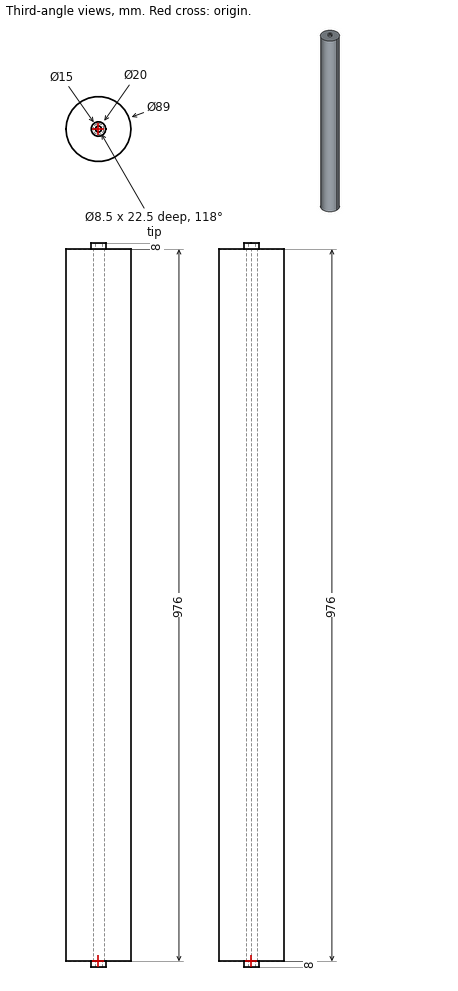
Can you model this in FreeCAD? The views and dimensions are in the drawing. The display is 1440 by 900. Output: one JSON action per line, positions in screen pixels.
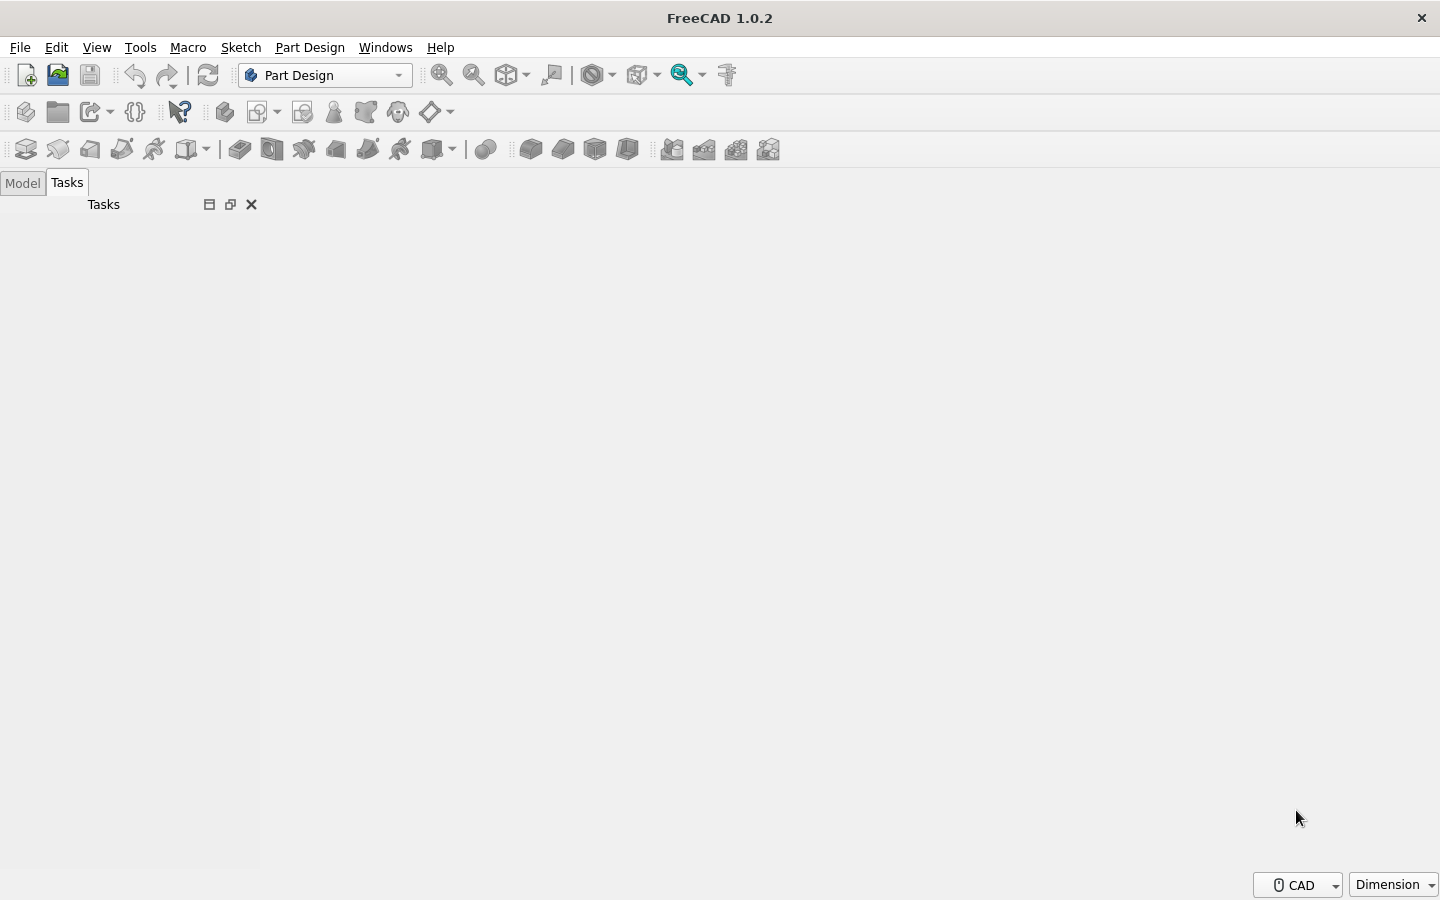
{"action": "left_click", "coordinate": [26, 76]}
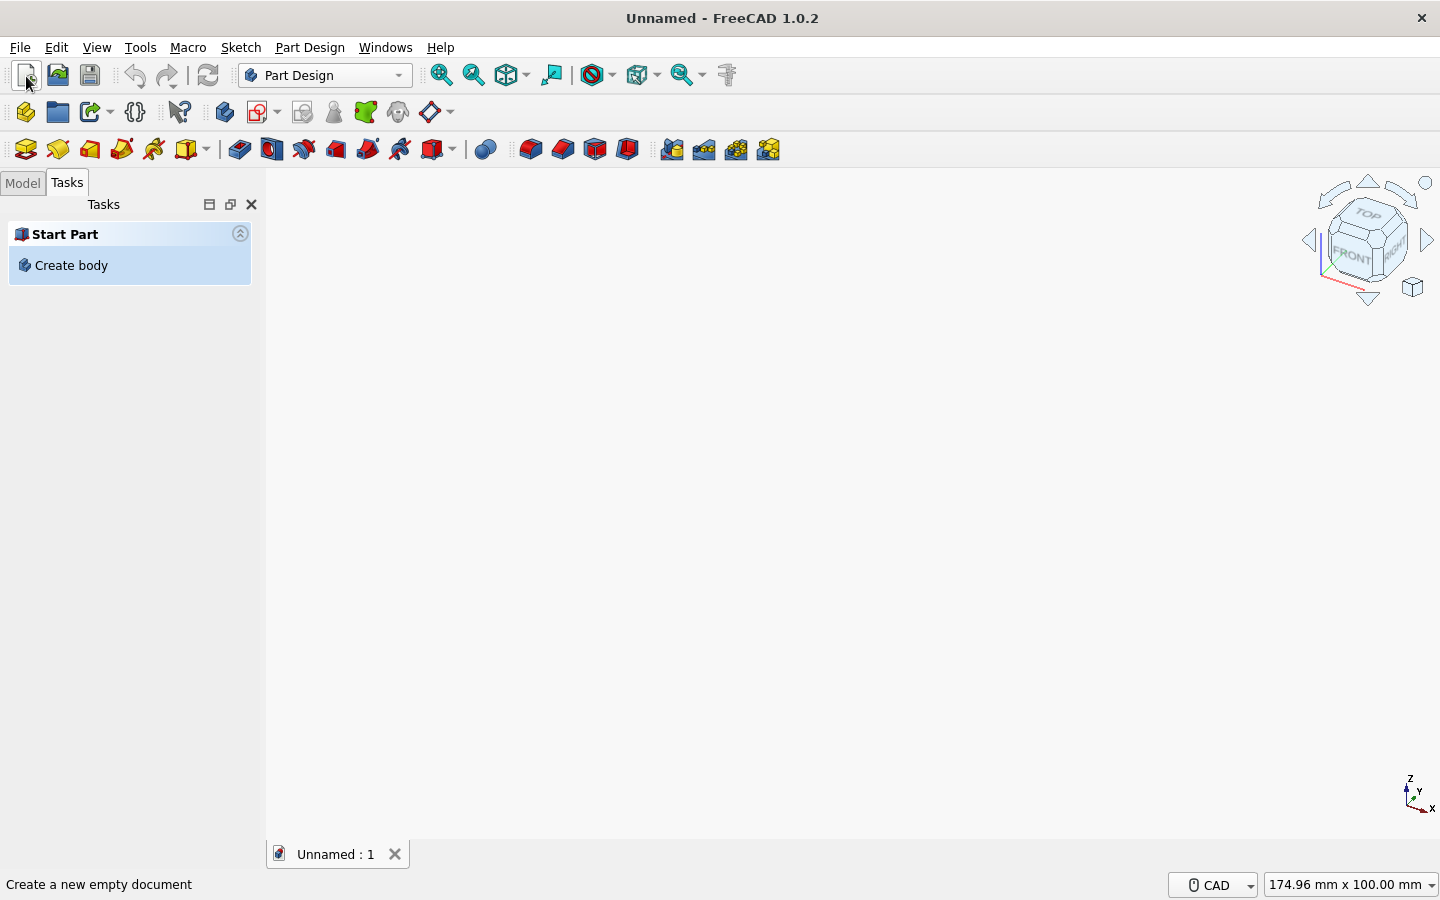
{"action": "left_click", "coordinate": [258, 112]}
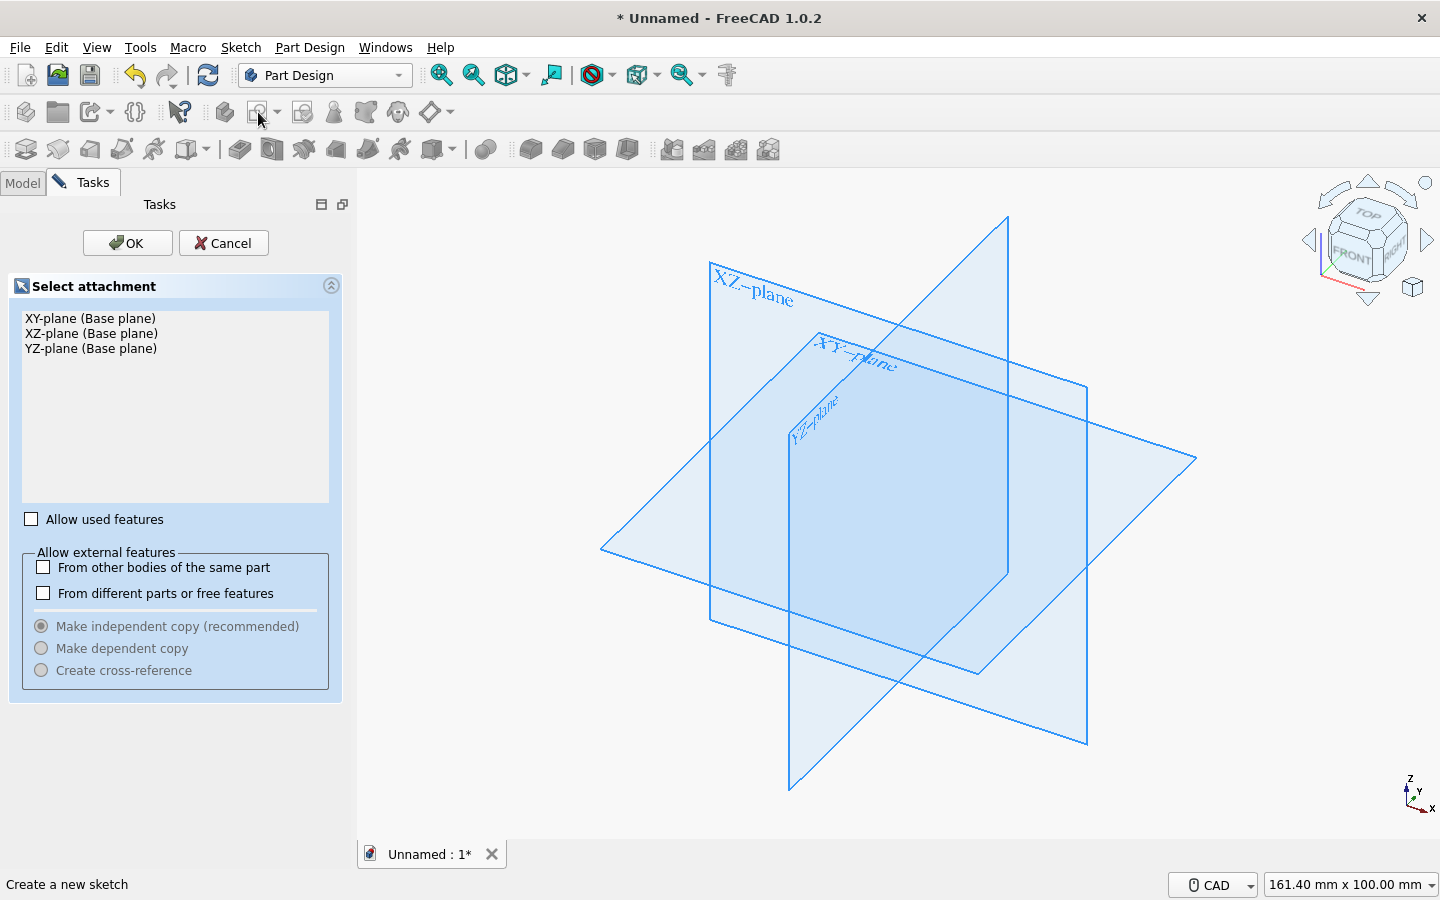
{"action": "left_click", "coordinate": [82, 318]}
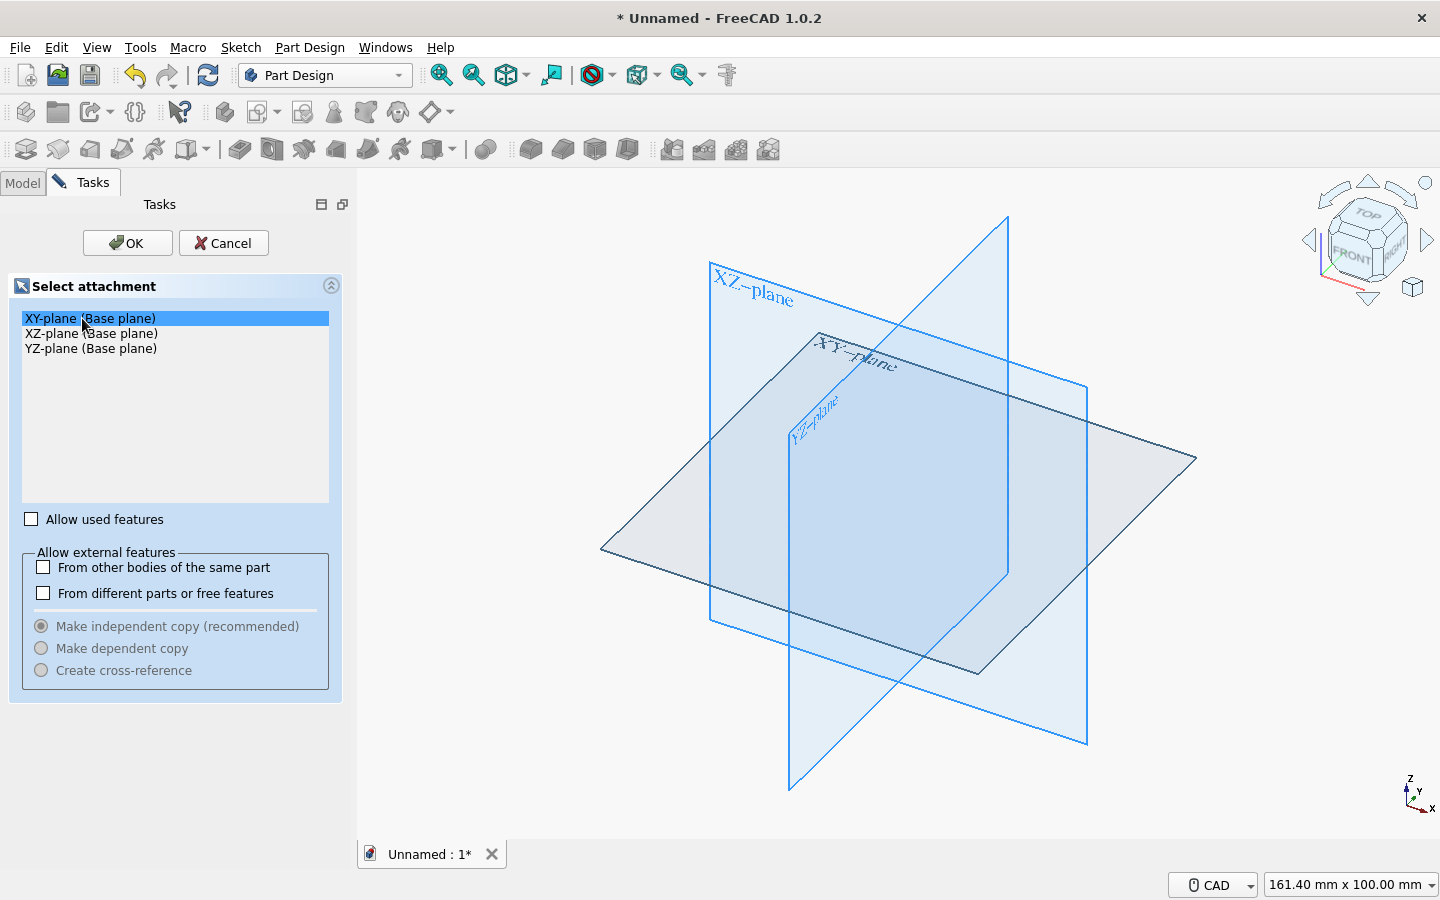
{"action": "left_click", "coordinate": [128, 243]}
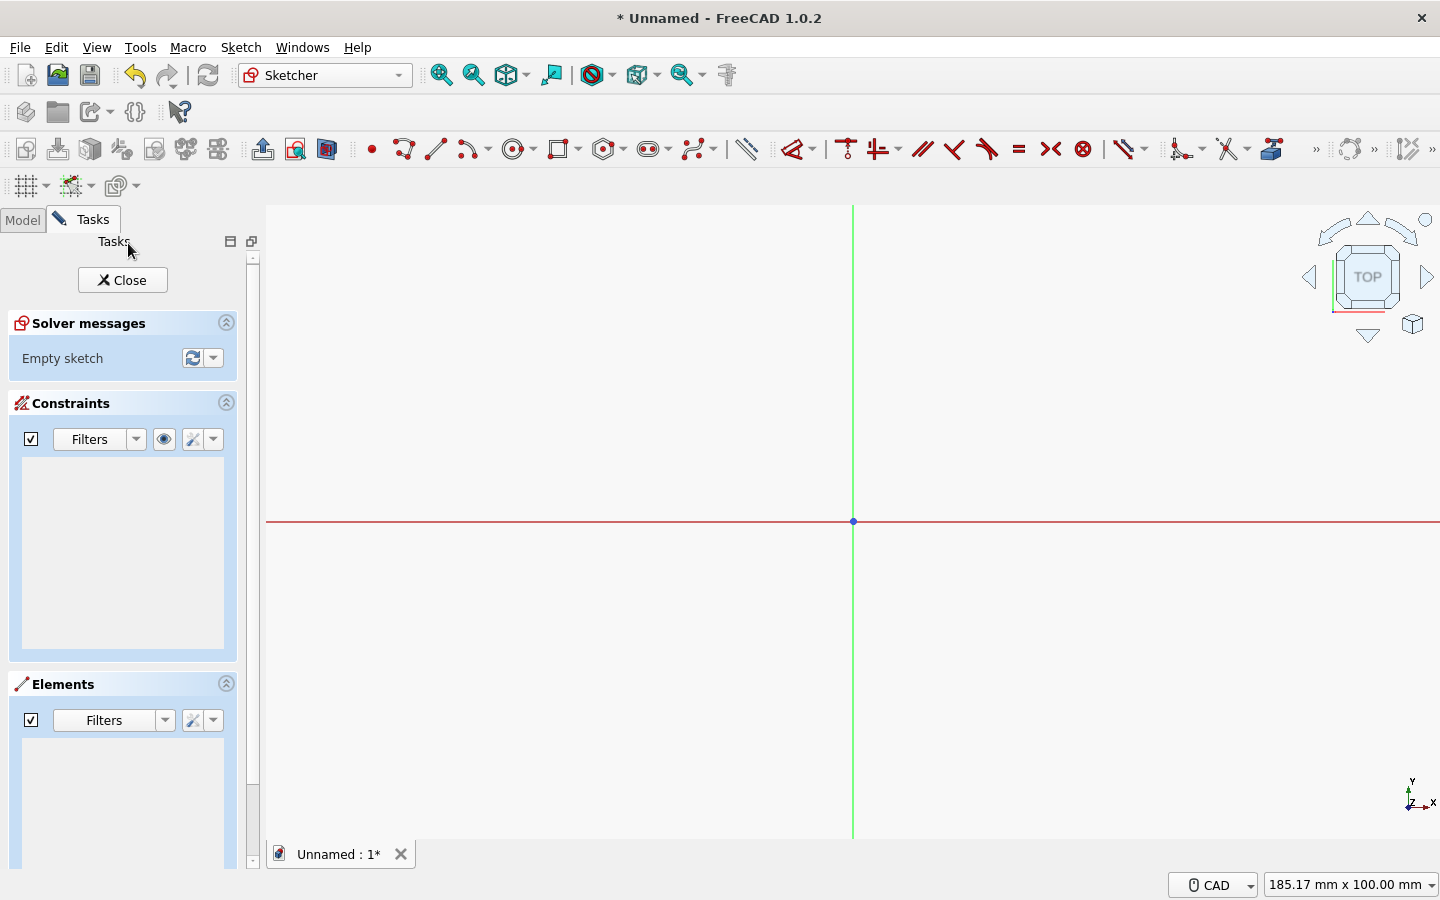
{"action": "scroll", "coordinate": [645, 522], "scroll_direction": "down", "scroll_amount": 2}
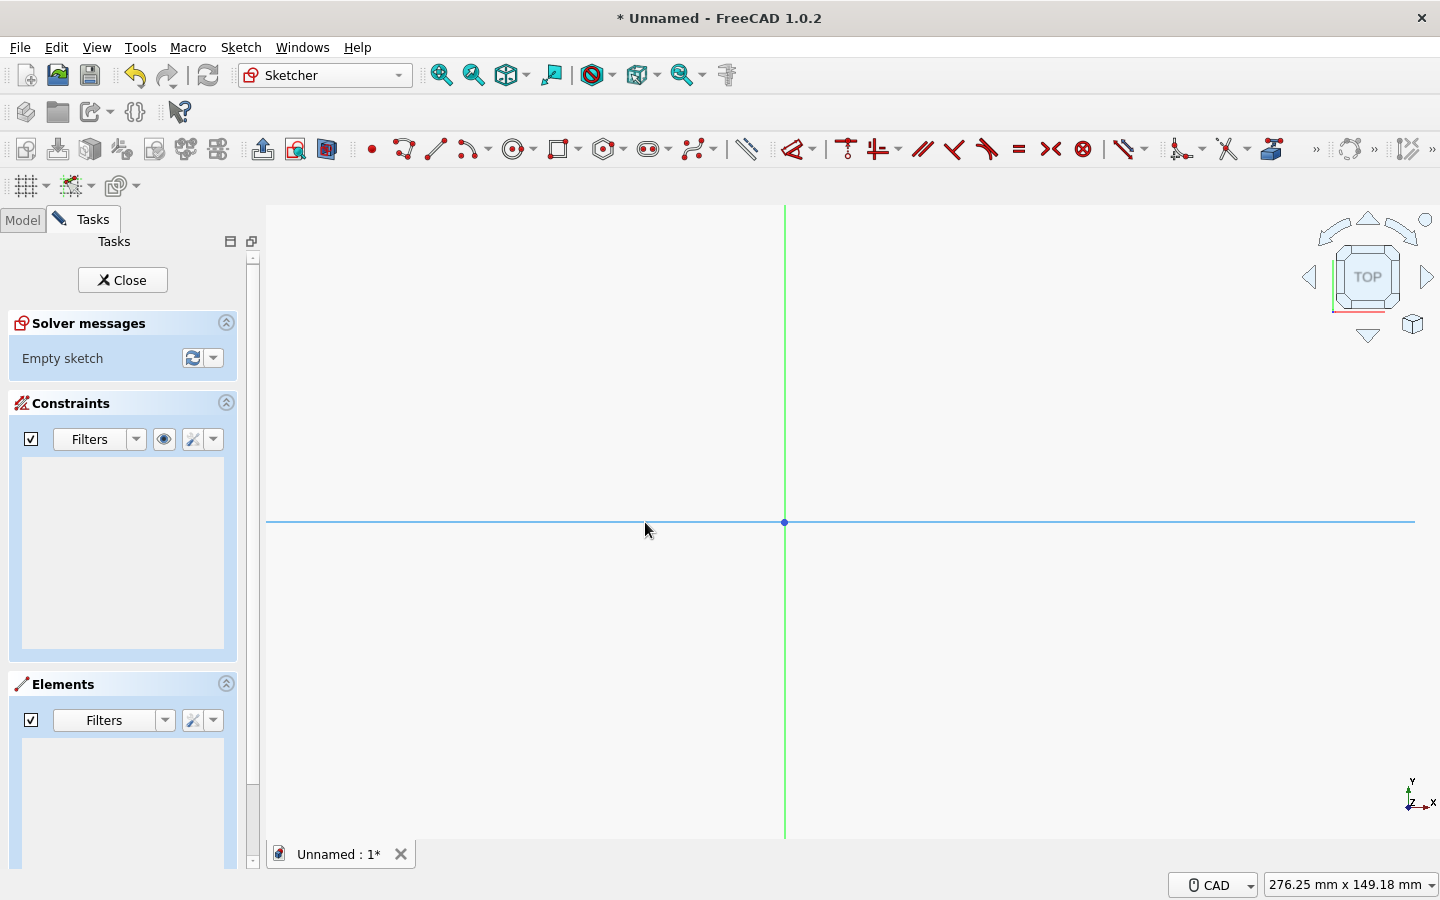
{"action": "left_click", "coordinate": [514, 150]}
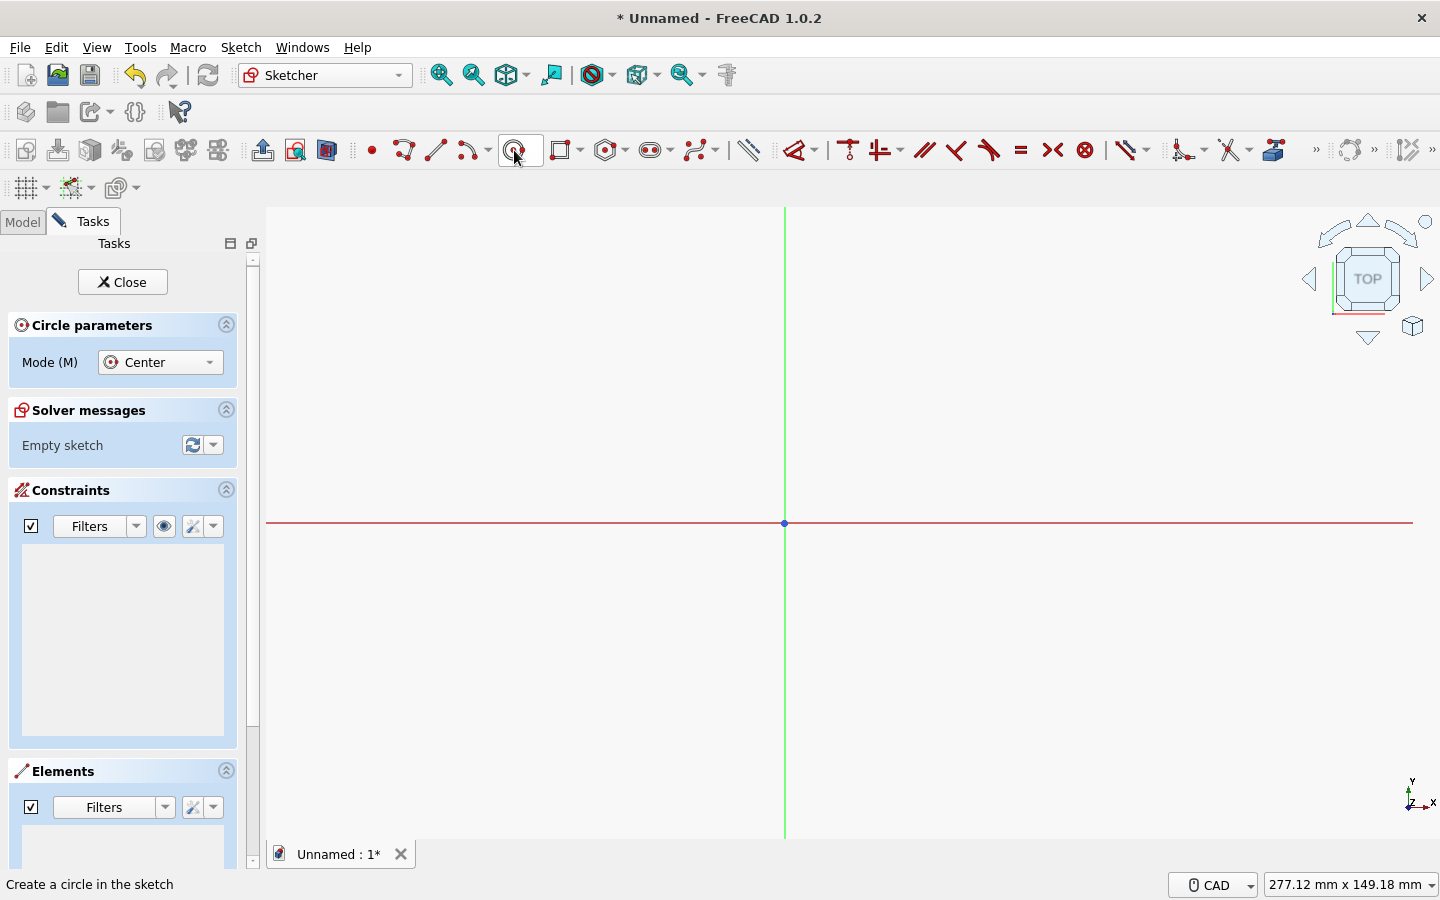
{"action": "left_click", "coordinate": [785, 523]}
{"action": "left_click", "coordinate": [918, 390]}
{"action": "key", "text": "Escape"}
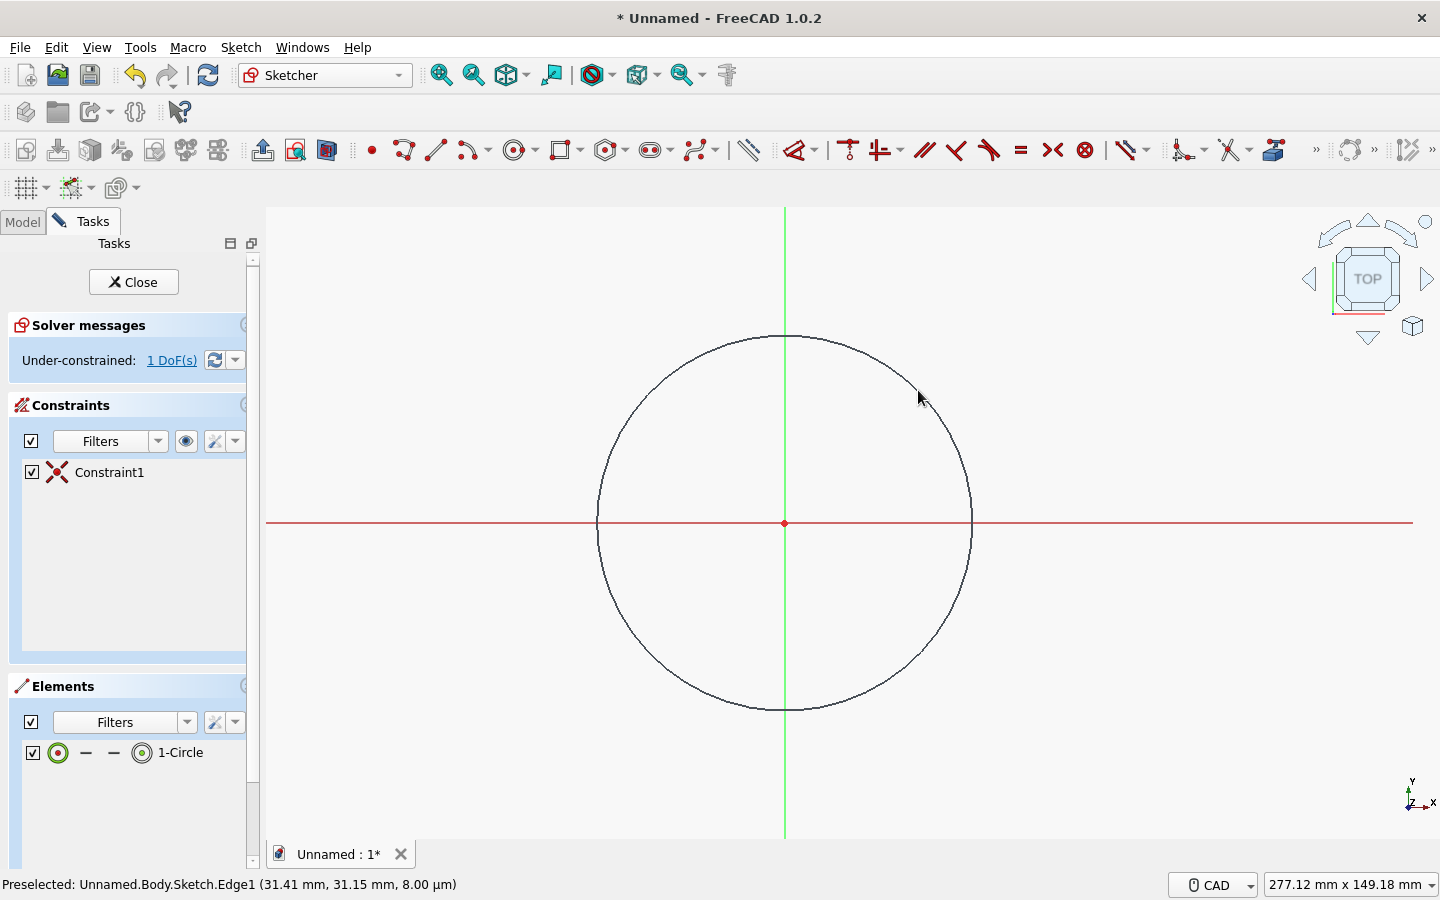
{"action": "left_click", "coordinate": [794, 150]}